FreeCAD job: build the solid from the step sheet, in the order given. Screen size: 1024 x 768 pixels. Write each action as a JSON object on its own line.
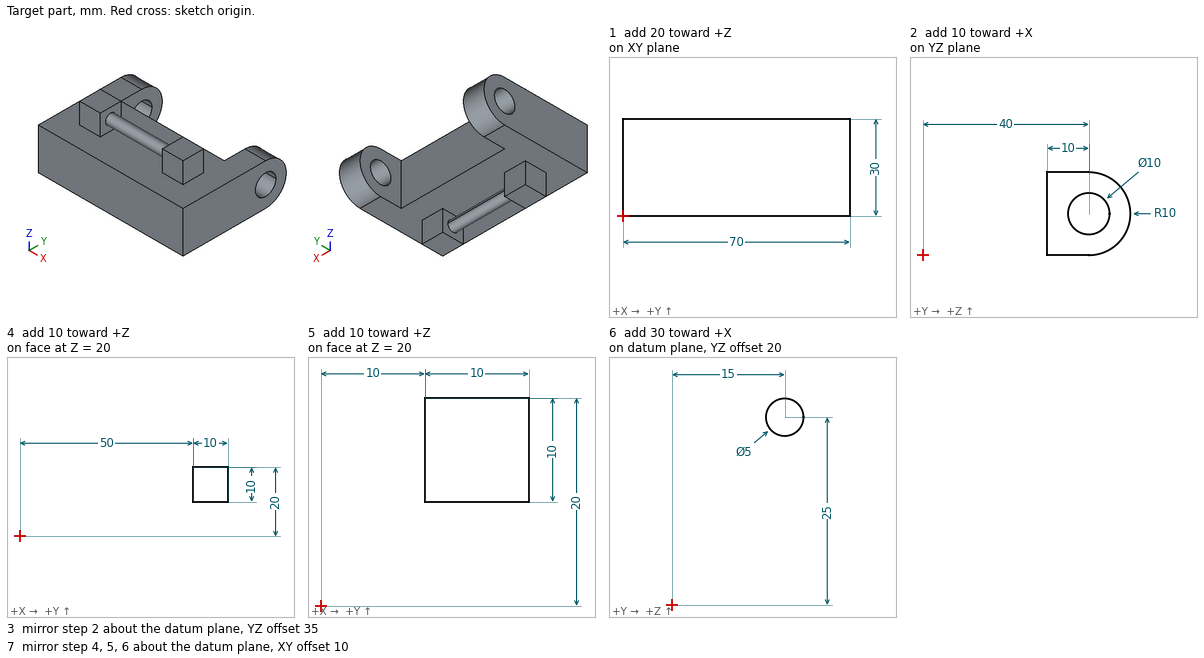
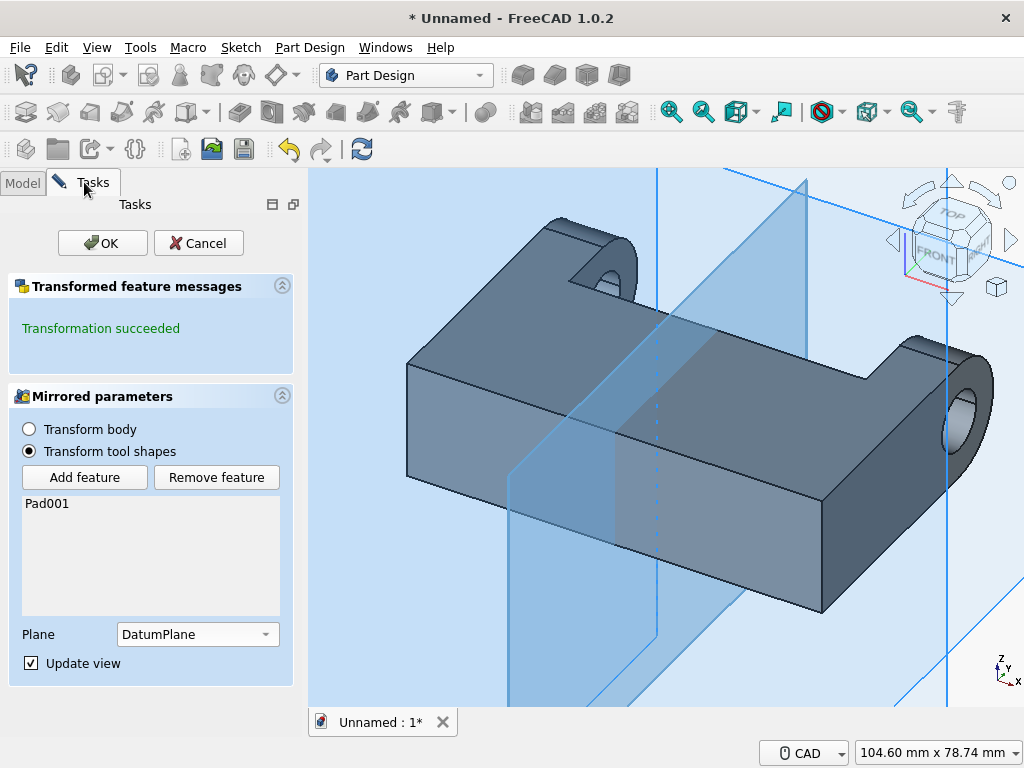
{"action": "left_click", "coordinate": [103, 243]}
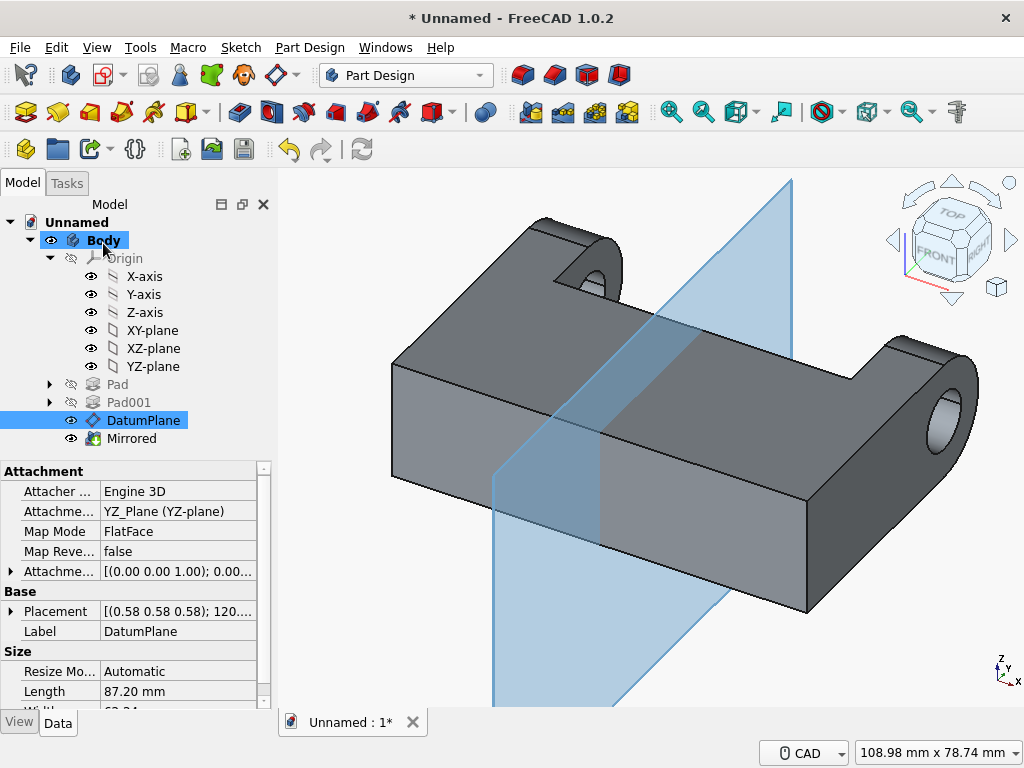
{"action": "left_click", "coordinate": [116, 420]}
{"action": "key", "text": "space"}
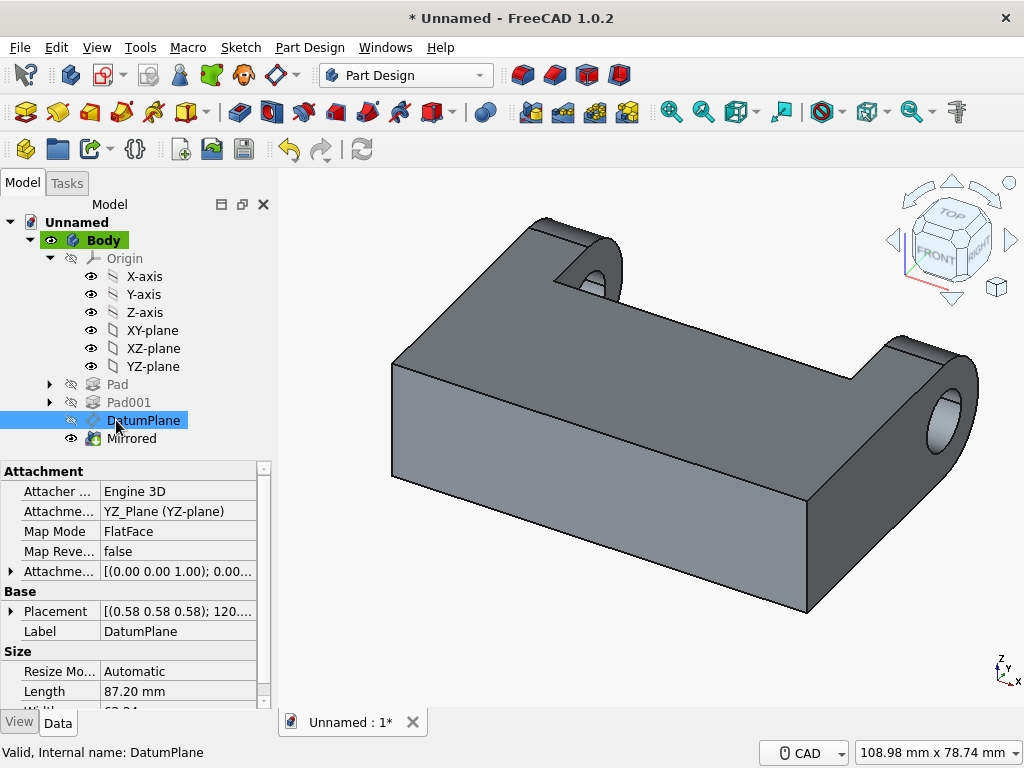
{"action": "left_click", "coordinate": [767, 422]}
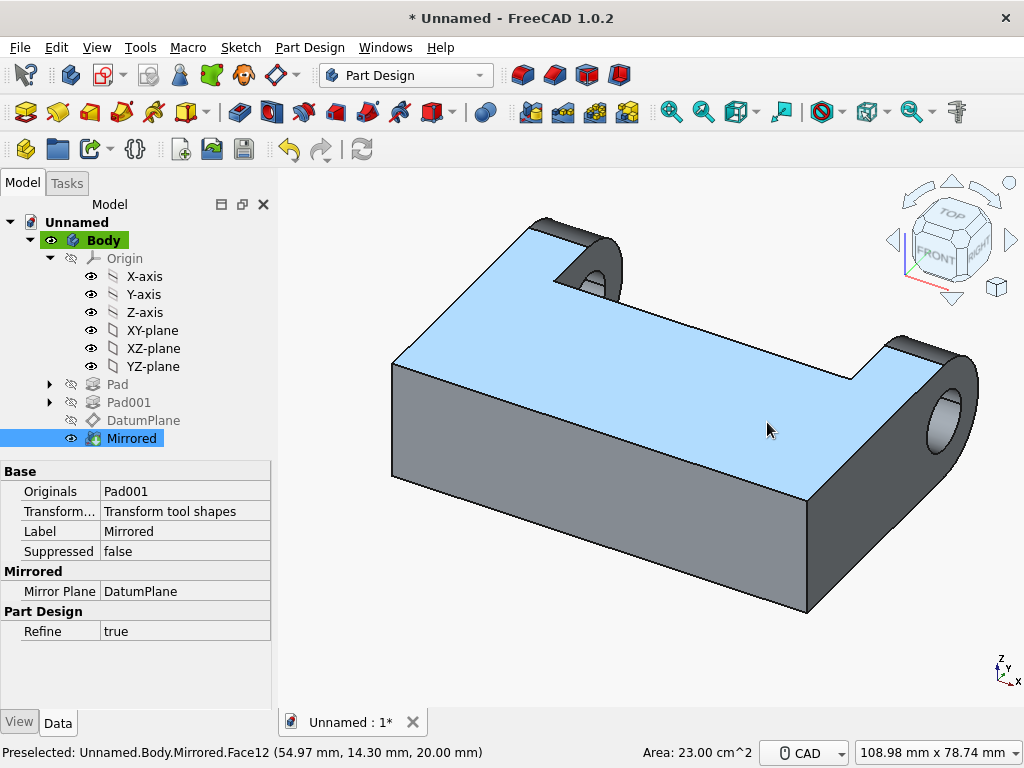
{"action": "left_click", "coordinate": [104, 76]}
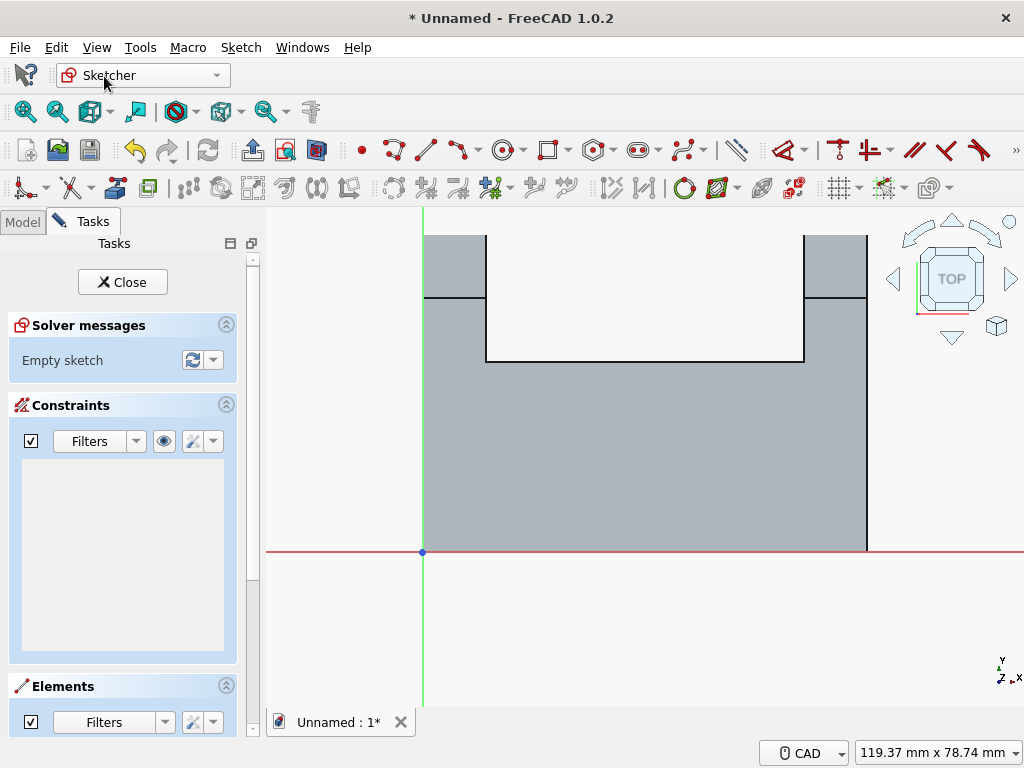
{"action": "scroll", "coordinate": [821, 457], "scroll_direction": "up", "scroll_amount": 8}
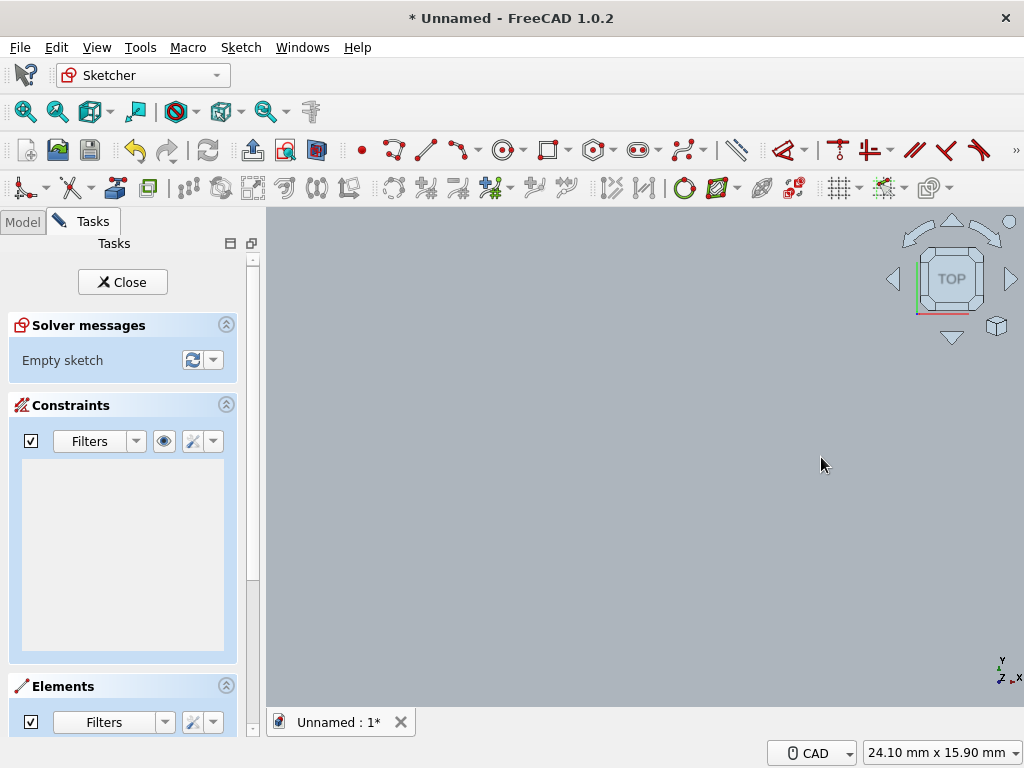
{"action": "key", "text": "g r"}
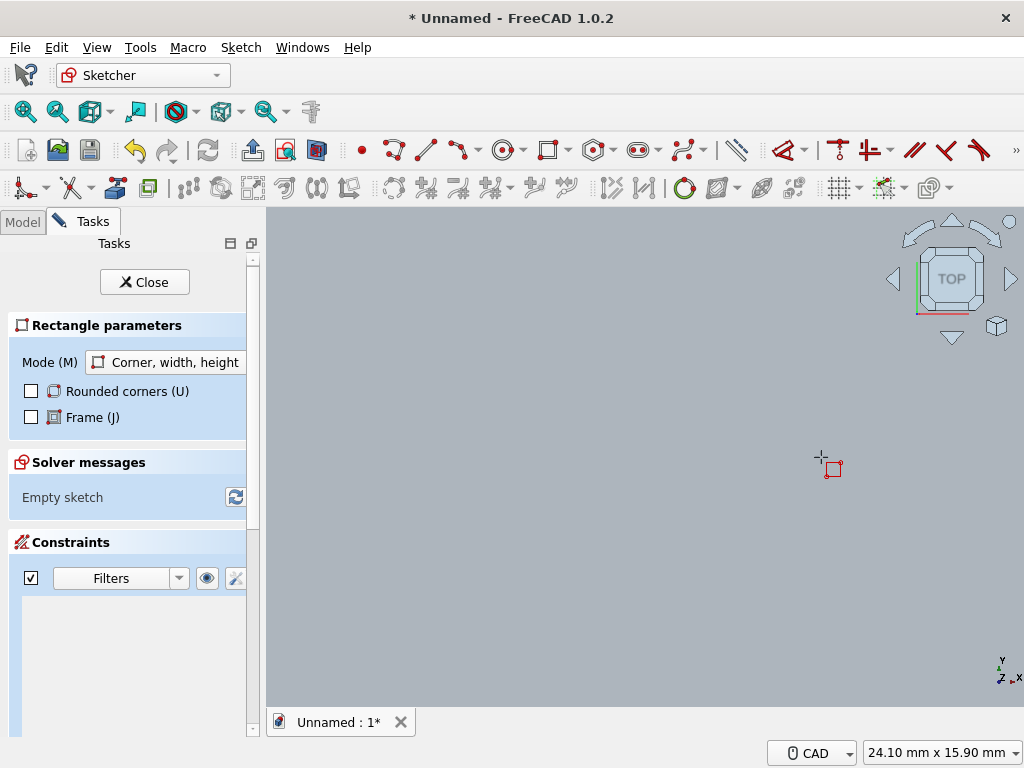
{"action": "left_click", "coordinate": [418, 298]}
{"action": "mouse_move", "coordinate": [733, 612]}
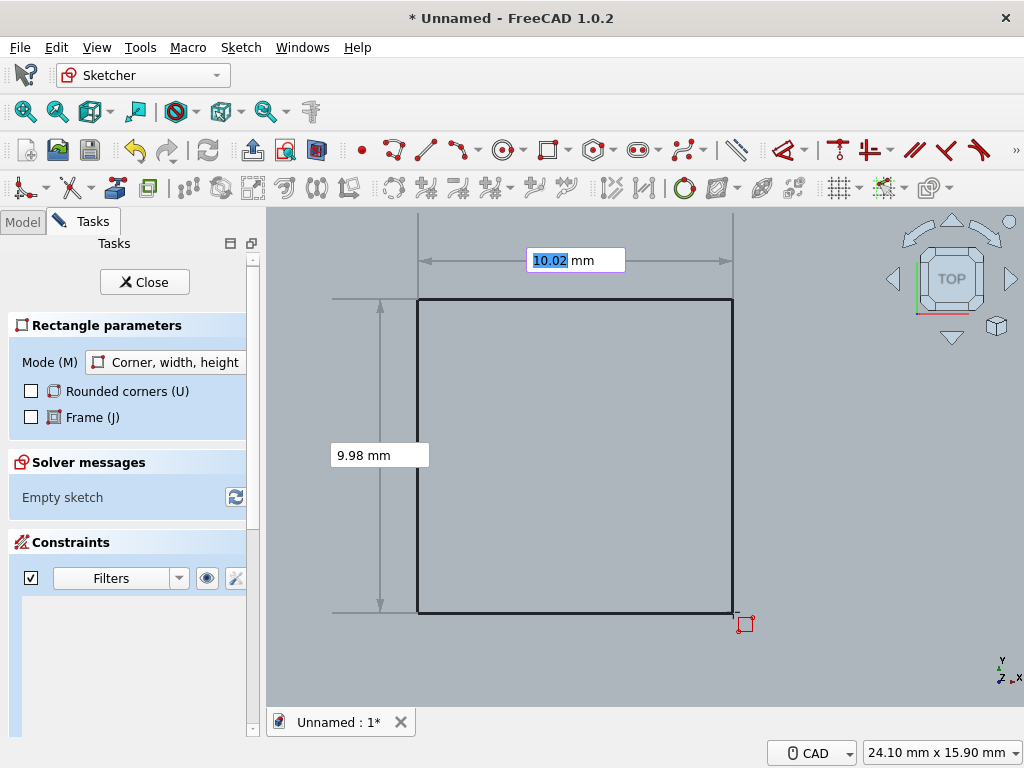
{"action": "type", "text": "10"}
{"action": "key", "text": "Tab"}
{"action": "type", "text": "10"}
{"action": "key", "text": "Return"}
{"action": "key", "text": "Escape"}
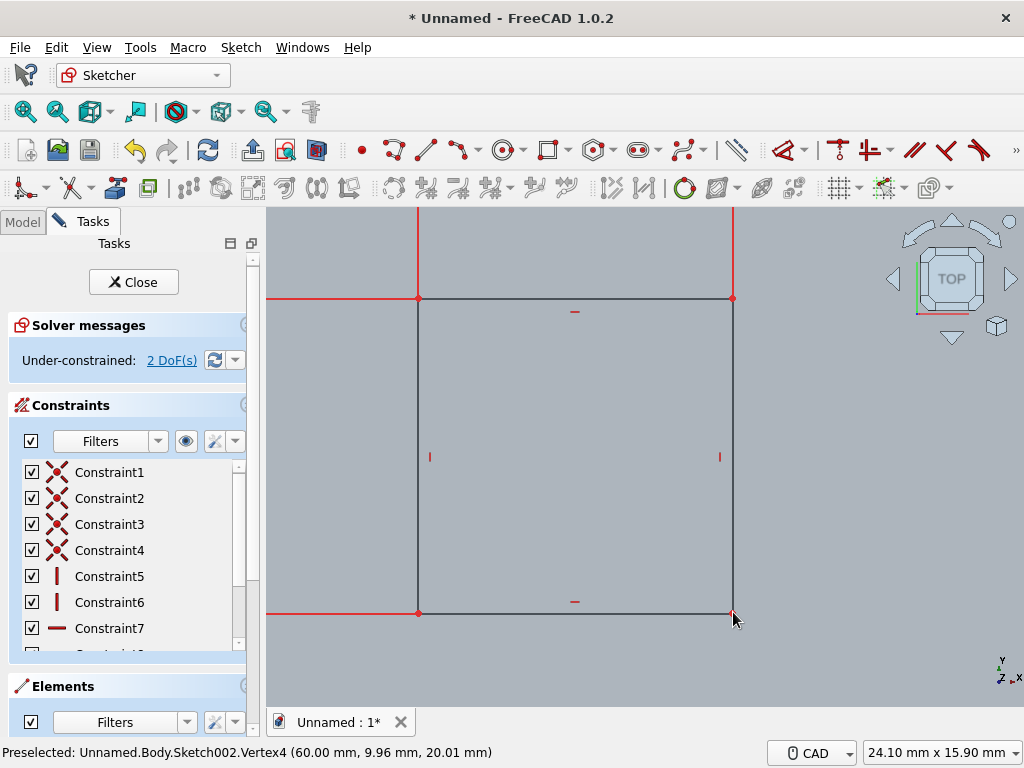
{"action": "left_click", "coordinate": [784, 150]}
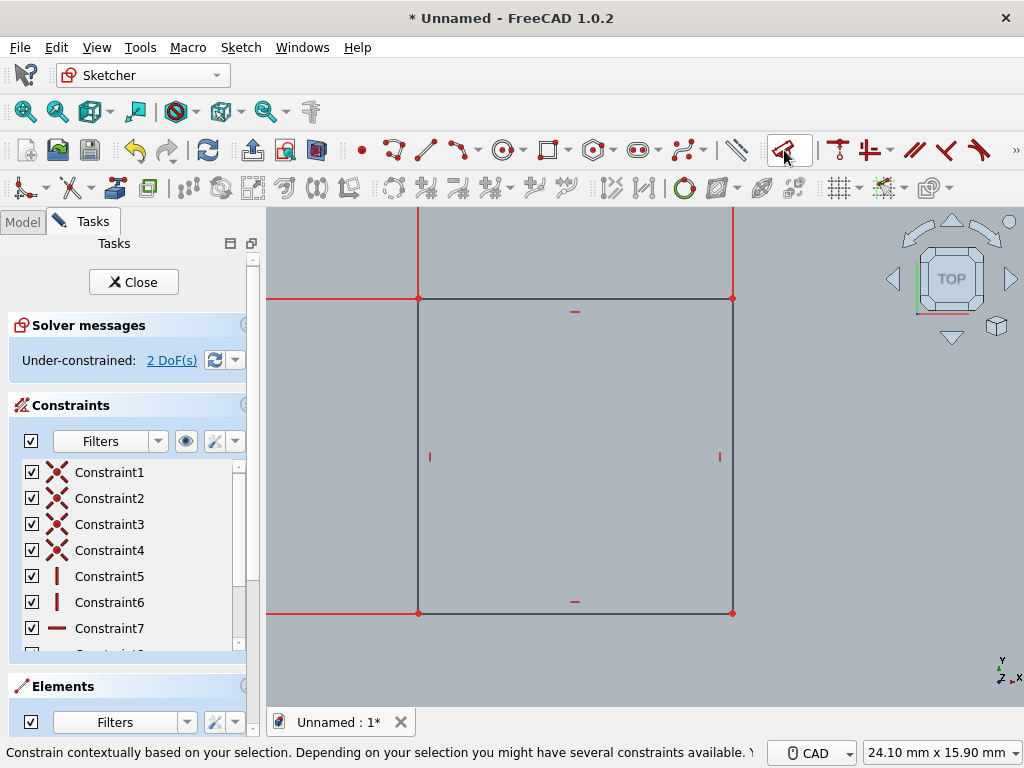
{"action": "left_click", "coordinate": [418, 299]}
{"action": "left_click", "coordinate": [356, 265]}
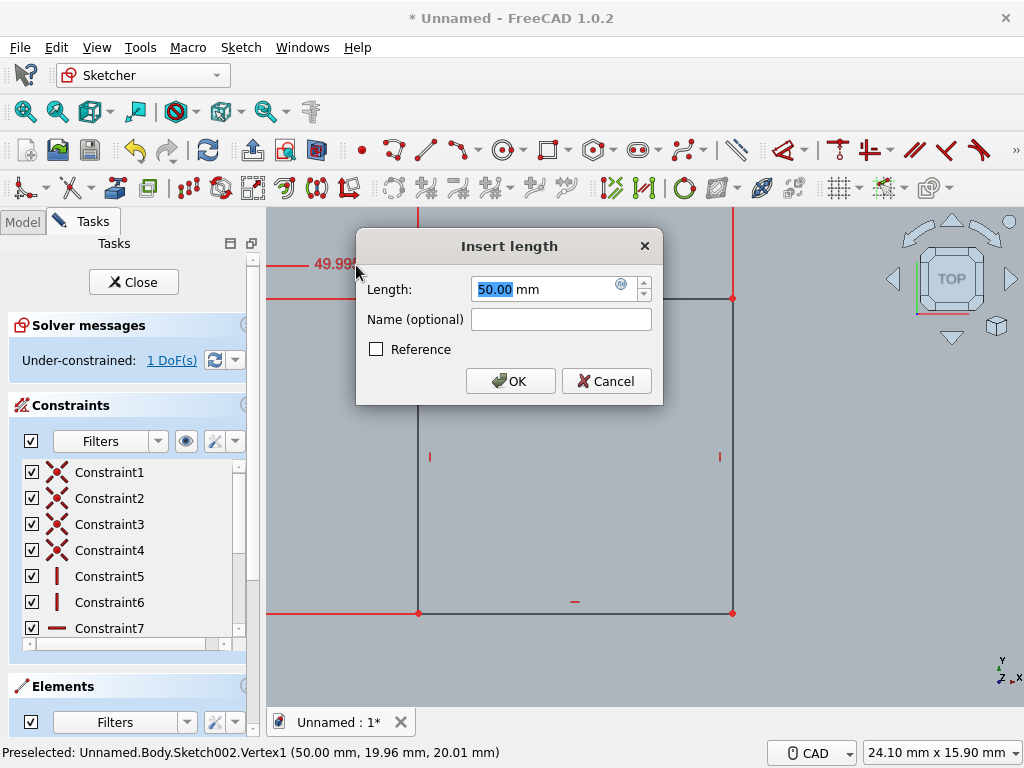
{"action": "type", "text": "50"}
{"action": "key", "text": "Return"}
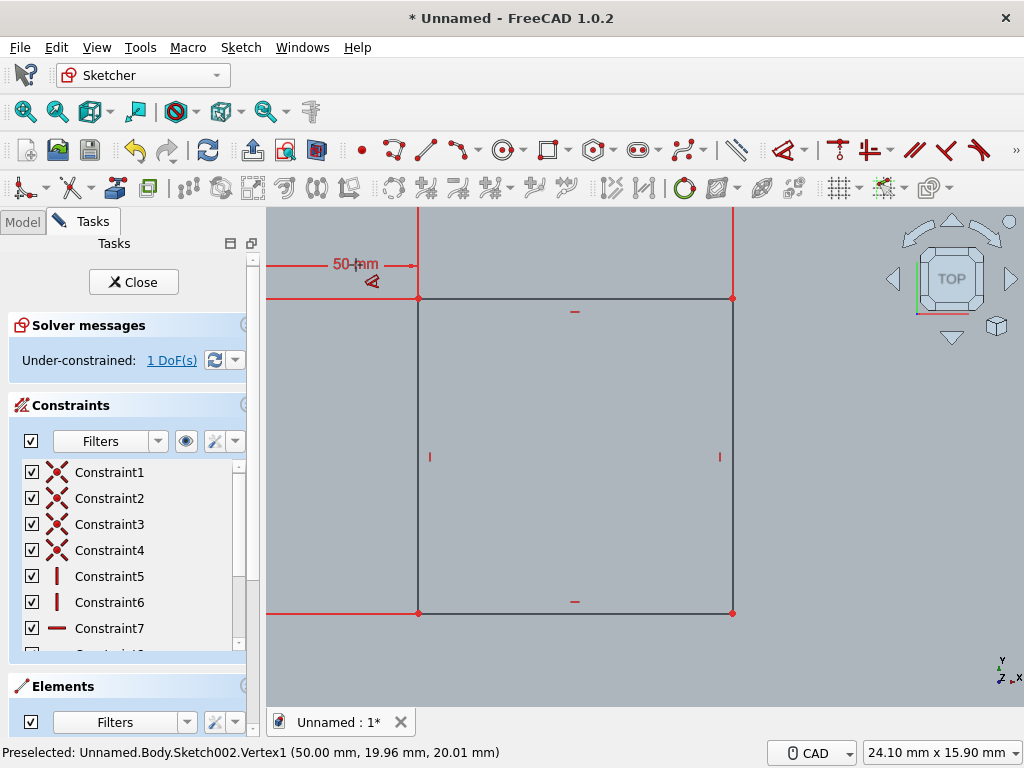
{"action": "left_click", "coordinate": [418, 299]}
{"action": "left_click", "coordinate": [452, 489]}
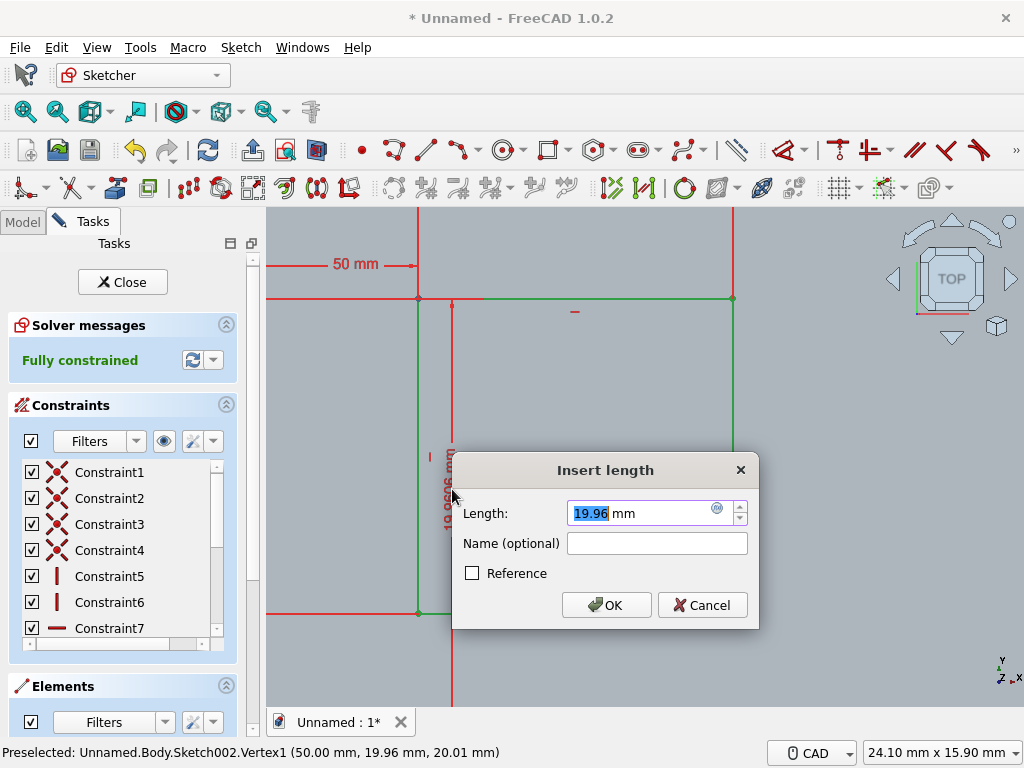
{"action": "type", "text": "20"}
{"action": "key", "text": "Return"}
{"action": "key", "text": "Escape"}